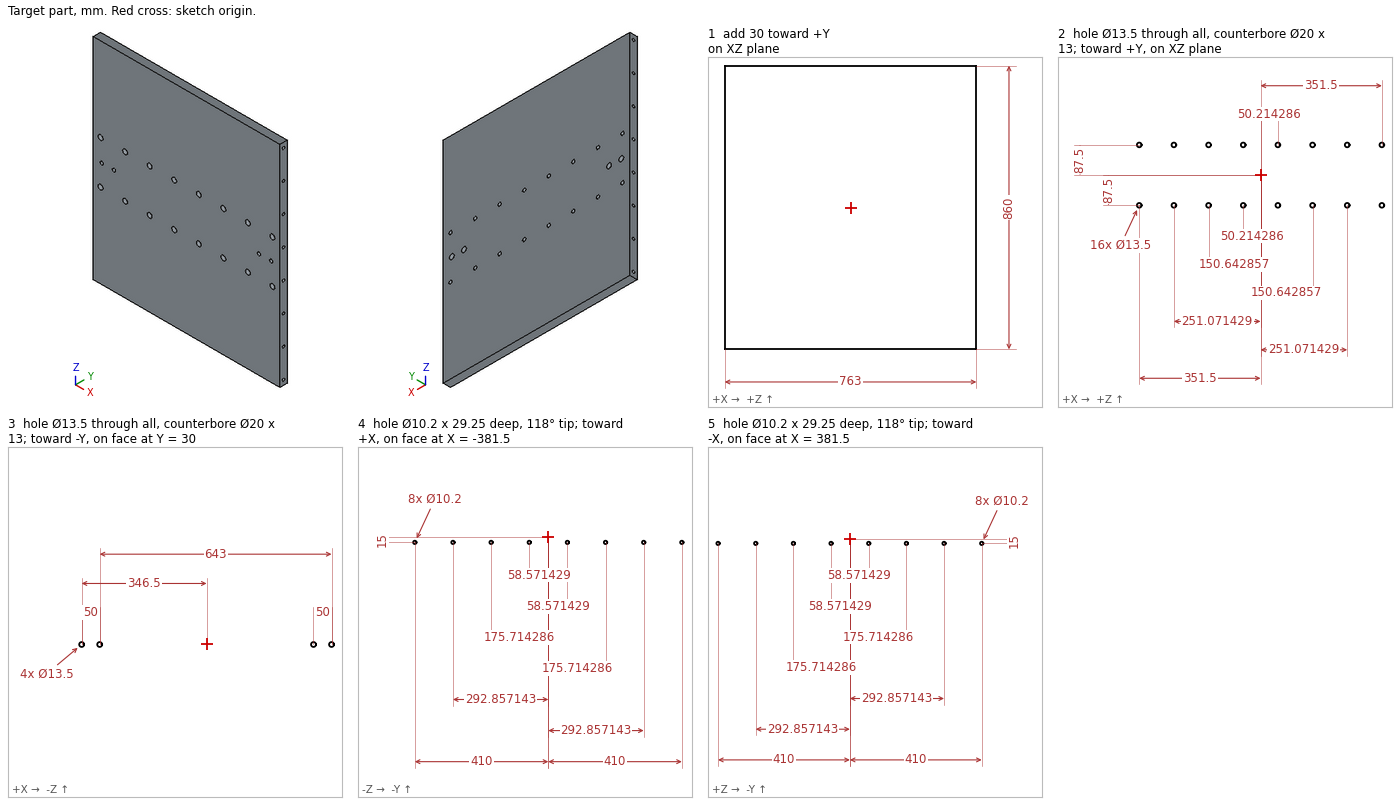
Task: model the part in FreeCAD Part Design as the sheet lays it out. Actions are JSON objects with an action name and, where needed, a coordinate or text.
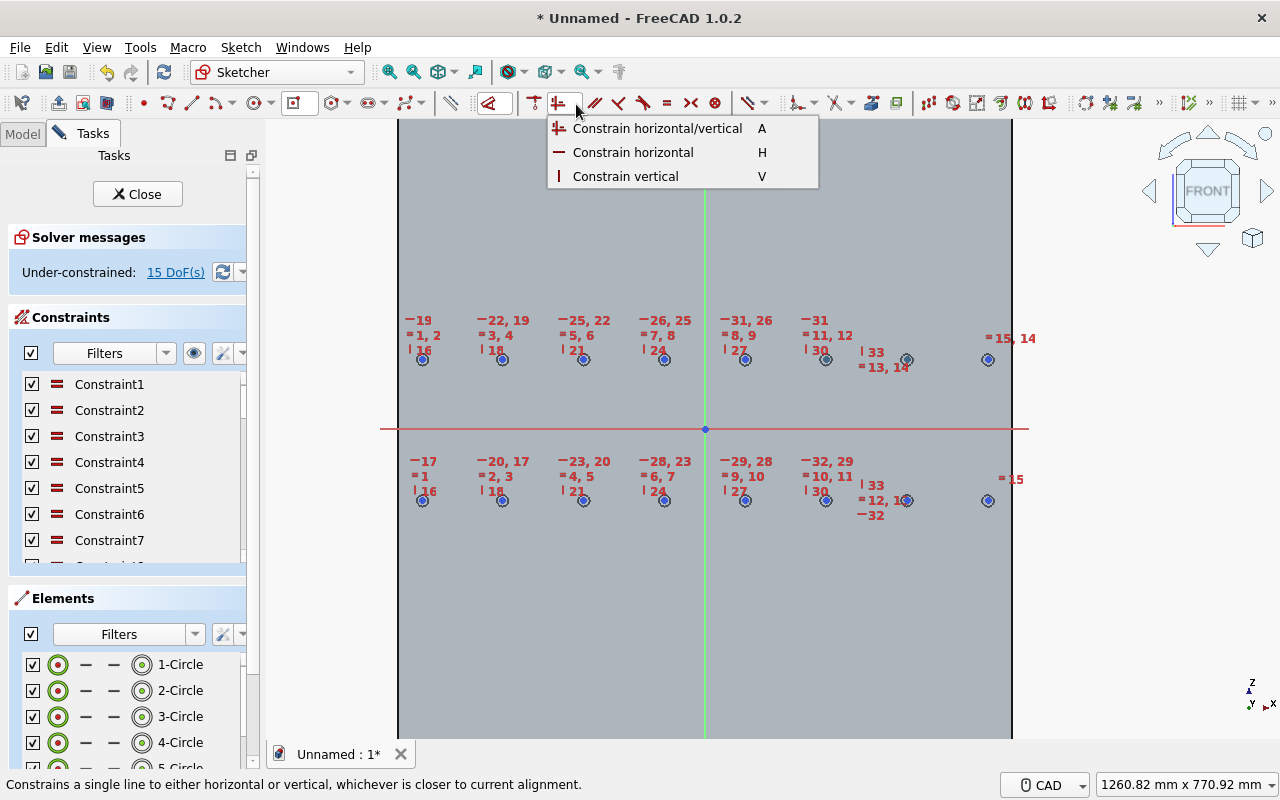
{"action": "left_click", "coordinate": [683, 152]}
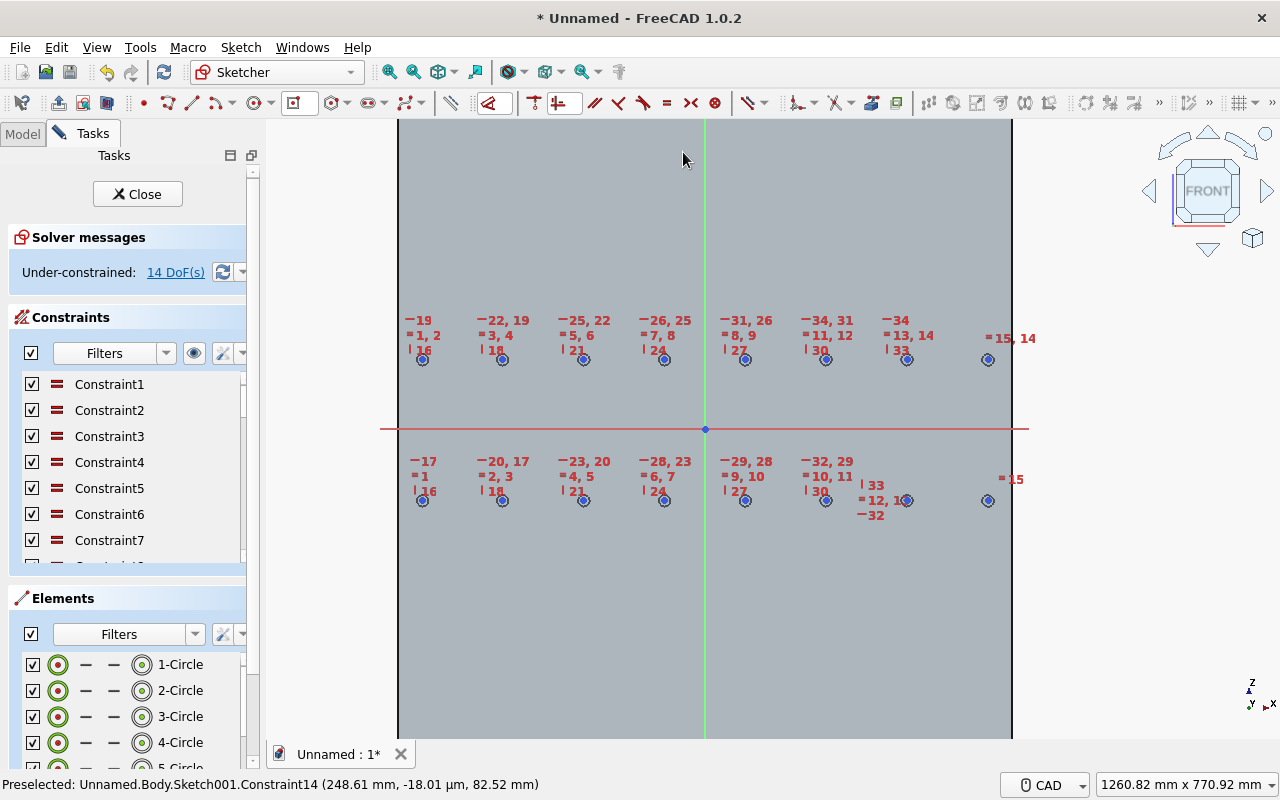
{"action": "left_click", "coordinate": [907, 360]}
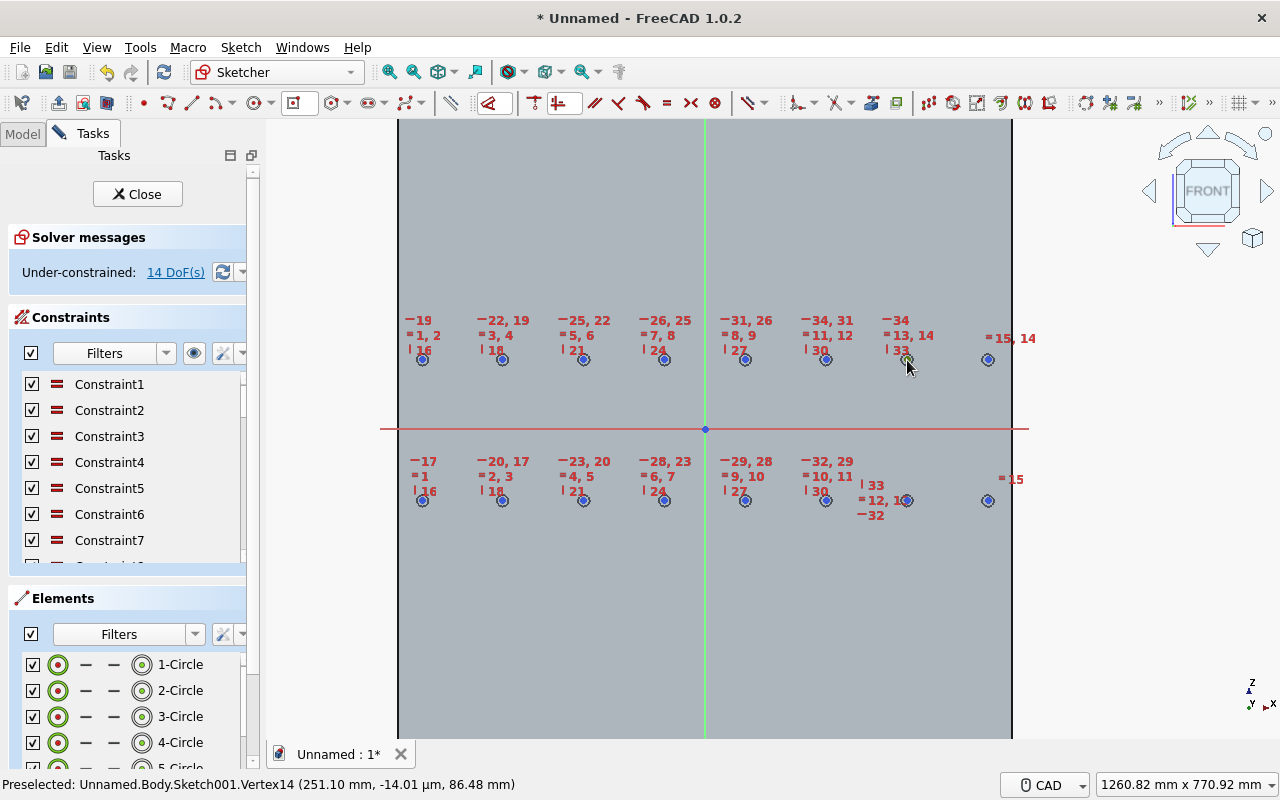
{"action": "left_click", "coordinate": [988, 360]}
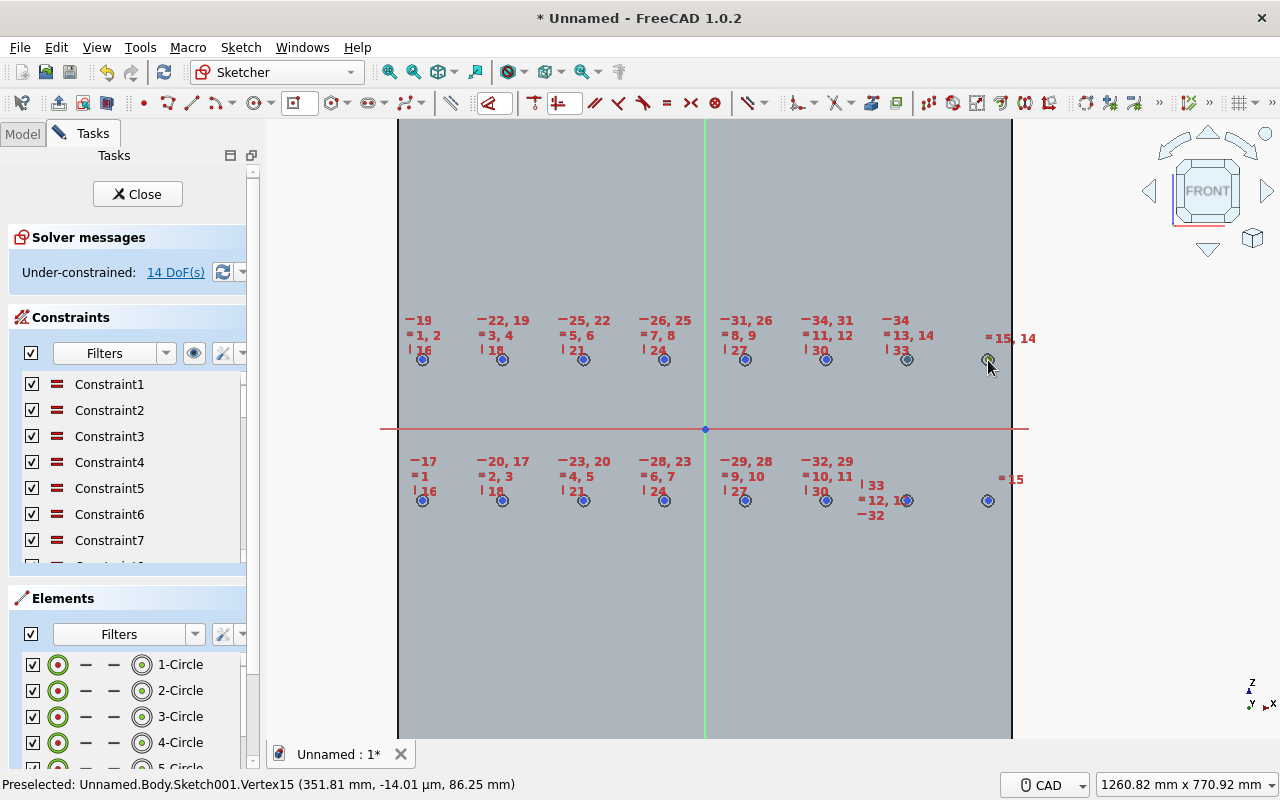
{"action": "key", "text": "h"}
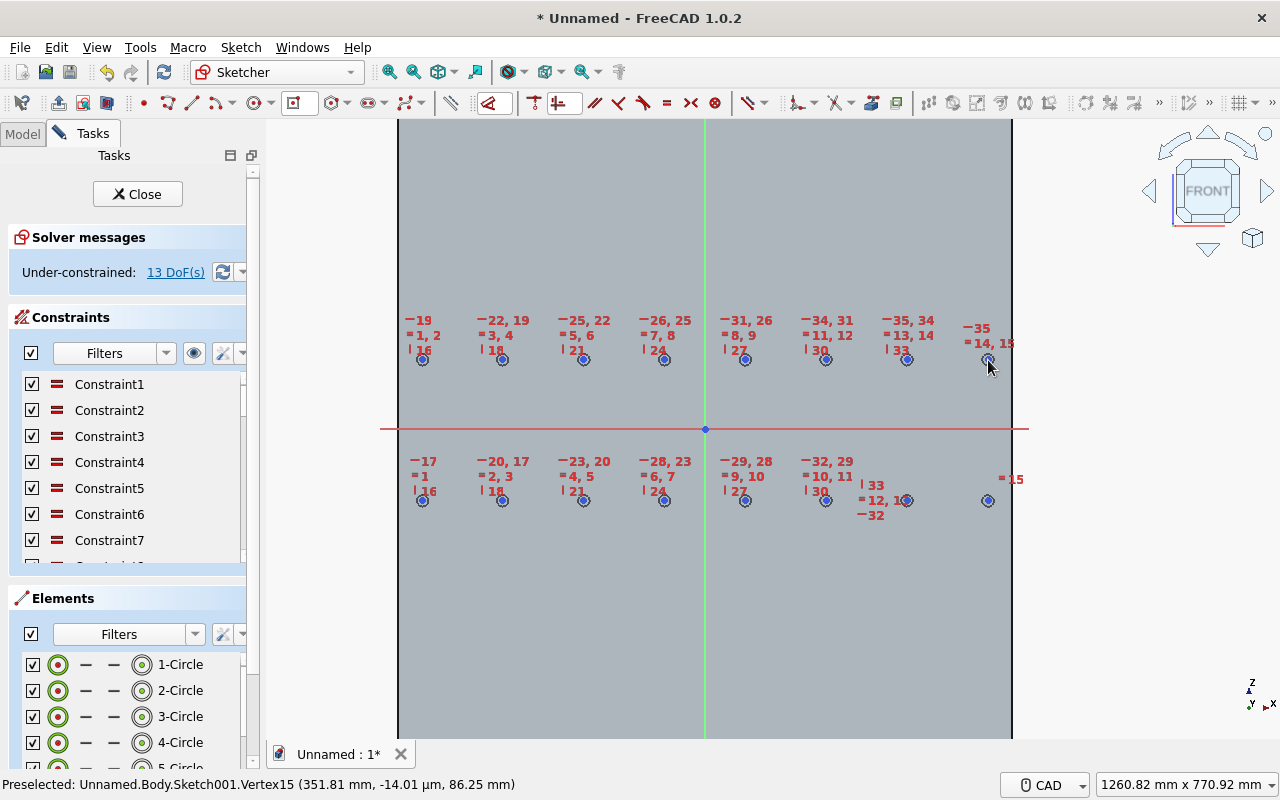
{"action": "left_click", "coordinate": [988, 360]}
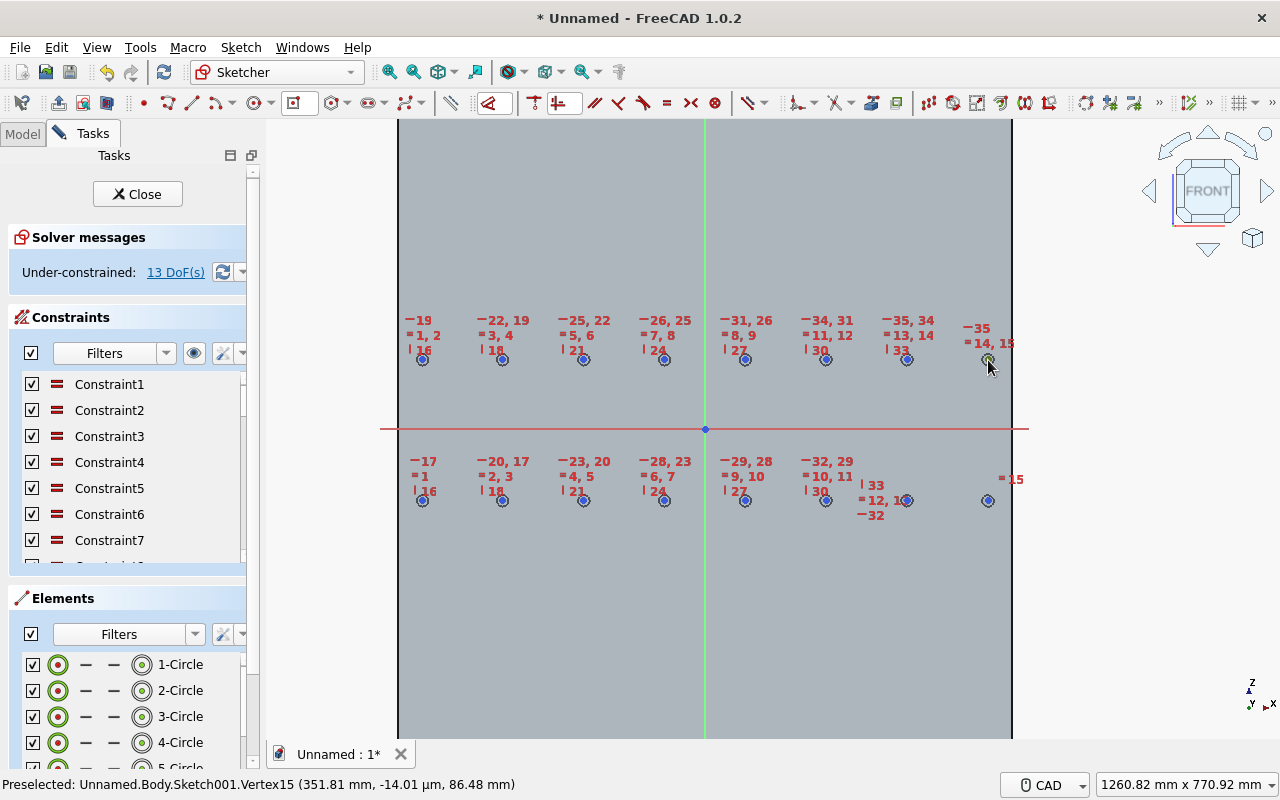
{"action": "left_click", "coordinate": [988, 501]}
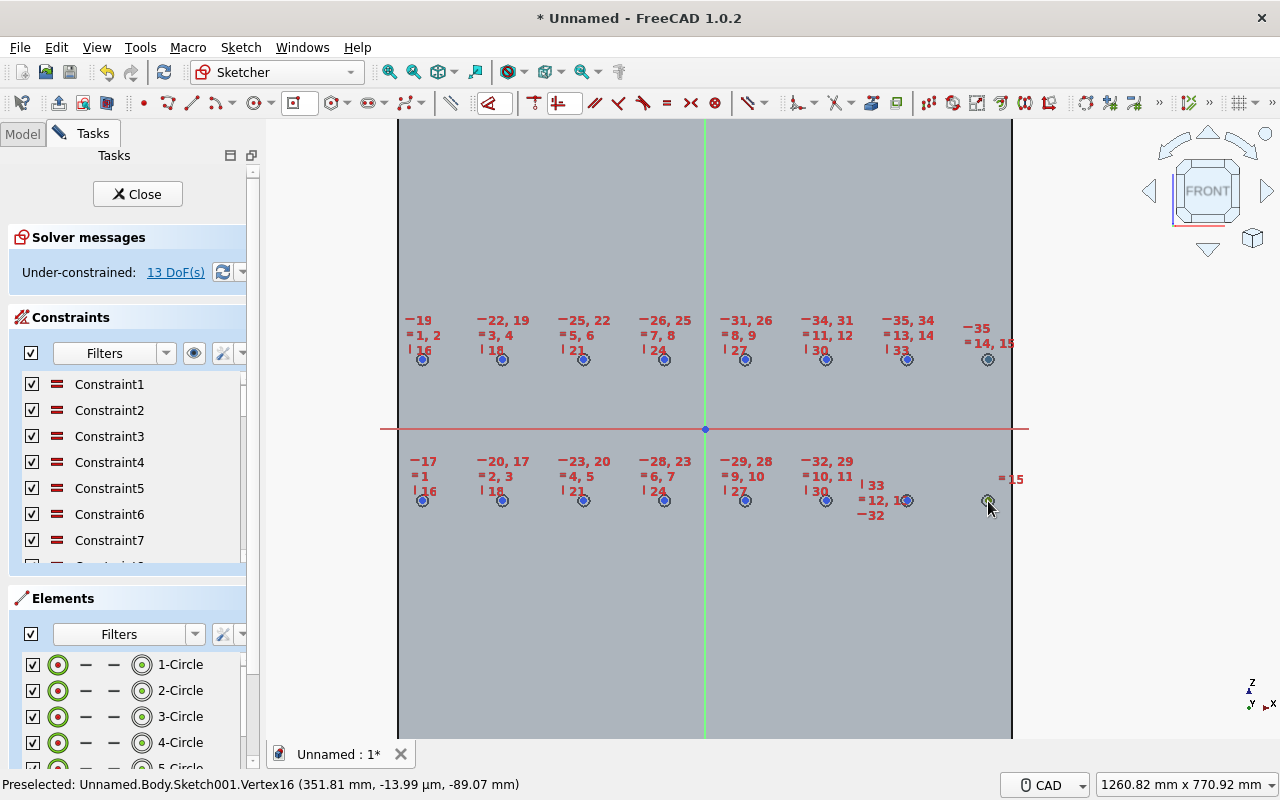
{"action": "left_click", "coordinate": [576, 104]}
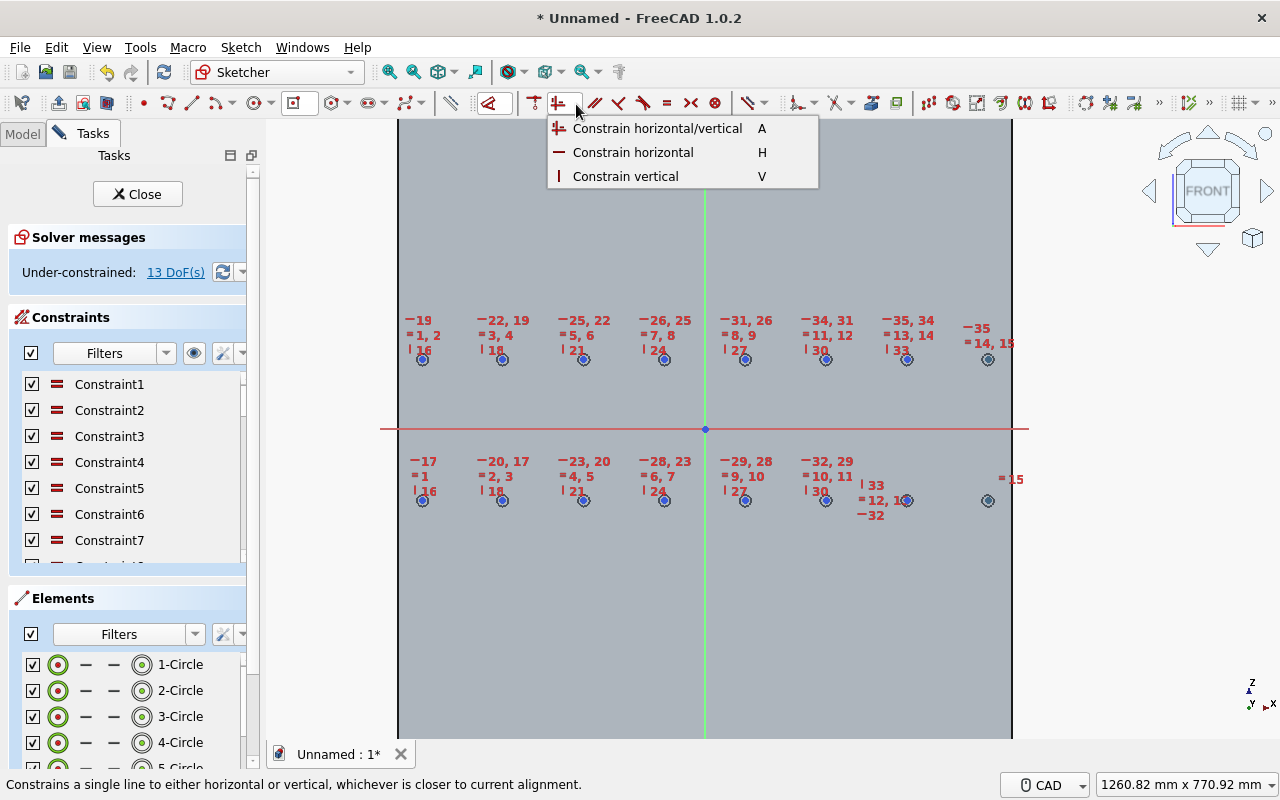
{"action": "left_click", "coordinate": [683, 176]}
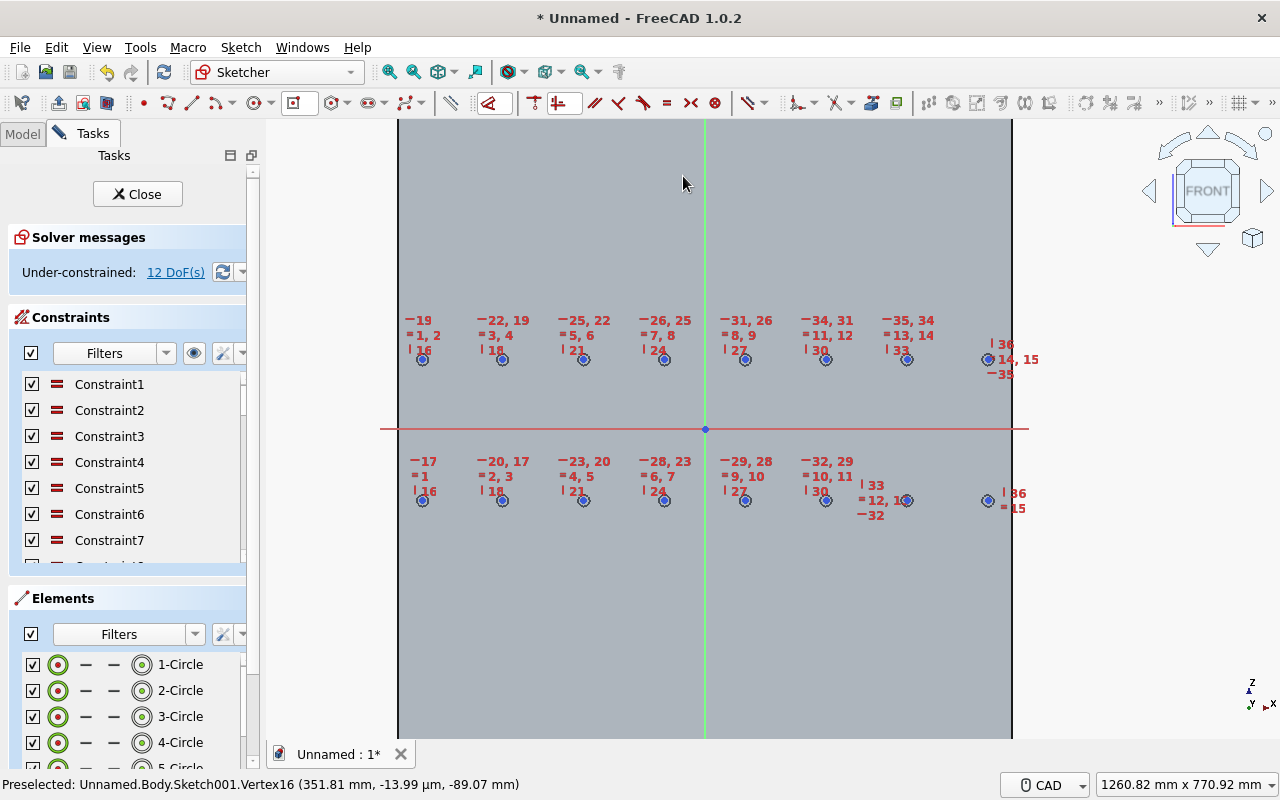
{"action": "left_click", "coordinate": [907, 501]}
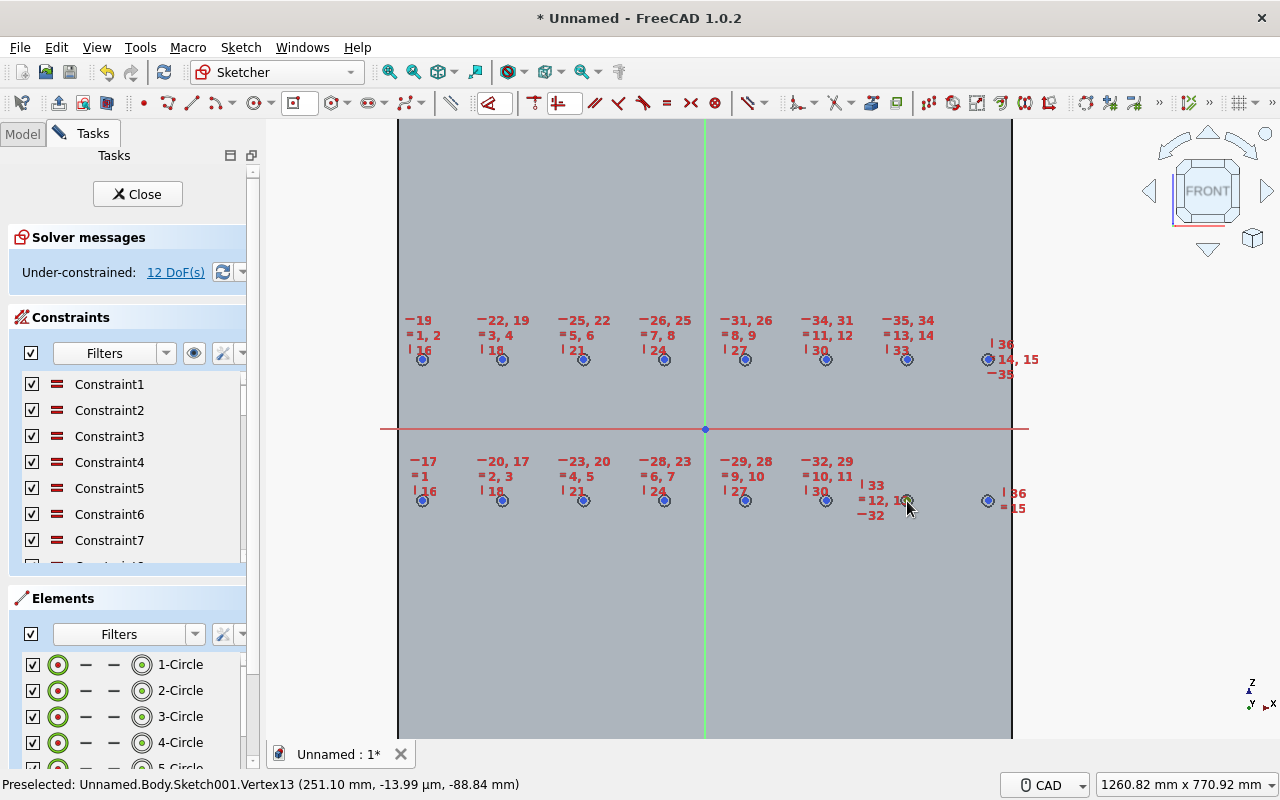
{"action": "left_click", "coordinate": [988, 501]}